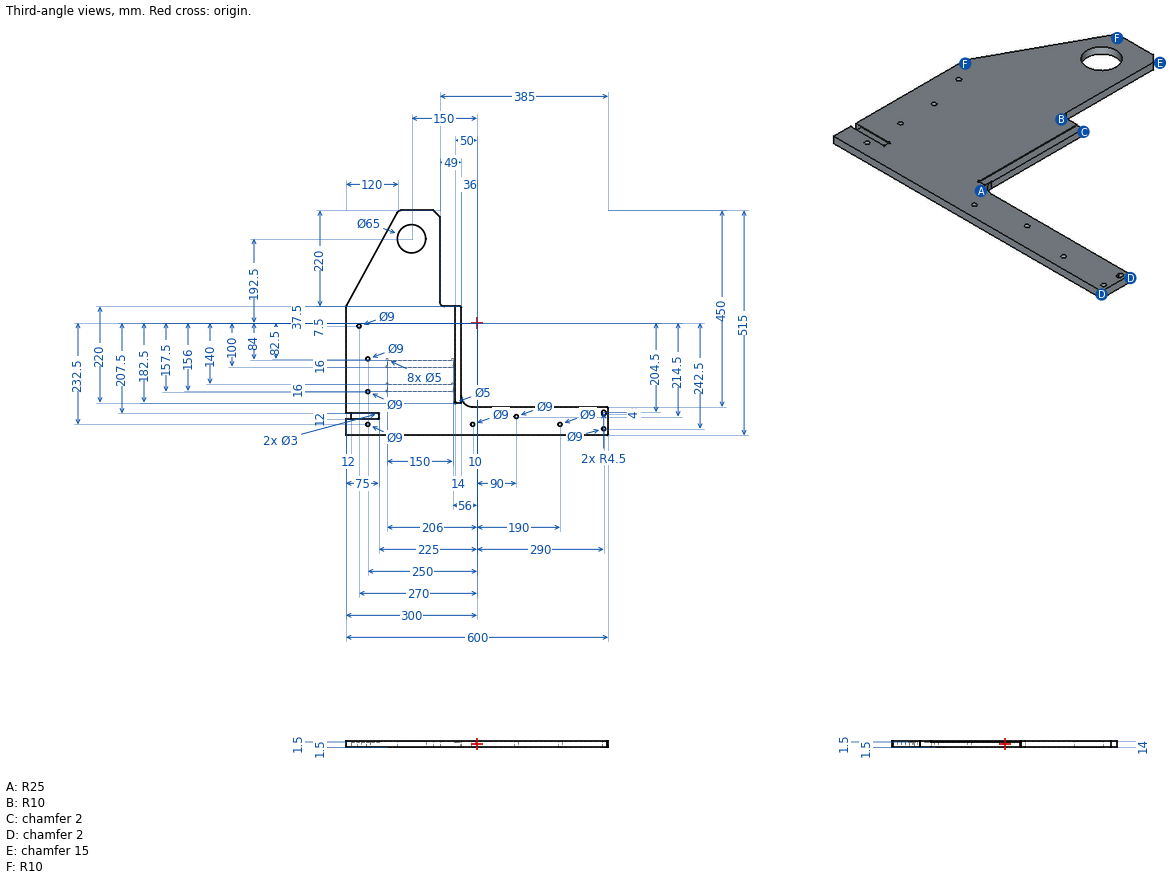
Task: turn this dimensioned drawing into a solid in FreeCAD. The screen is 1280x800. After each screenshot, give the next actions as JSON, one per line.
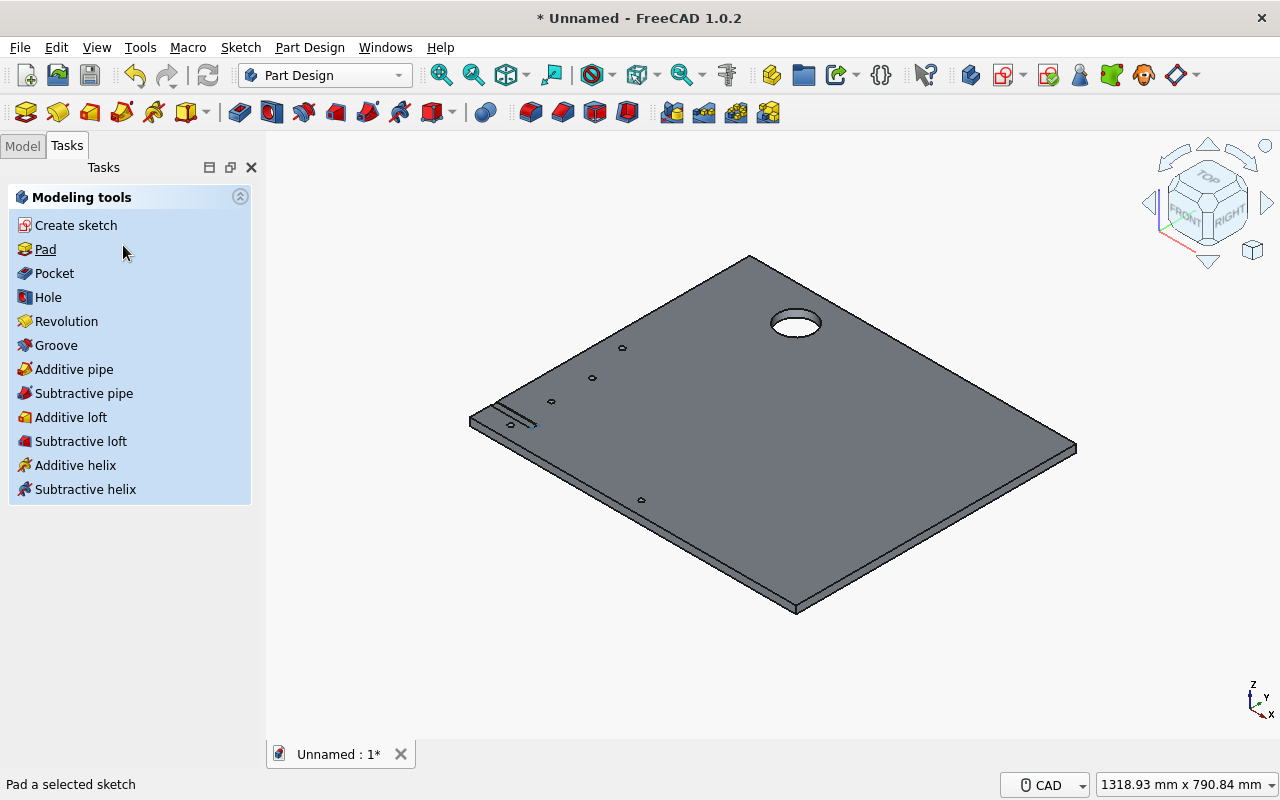
{"action": "left_click", "coordinate": [240, 112]}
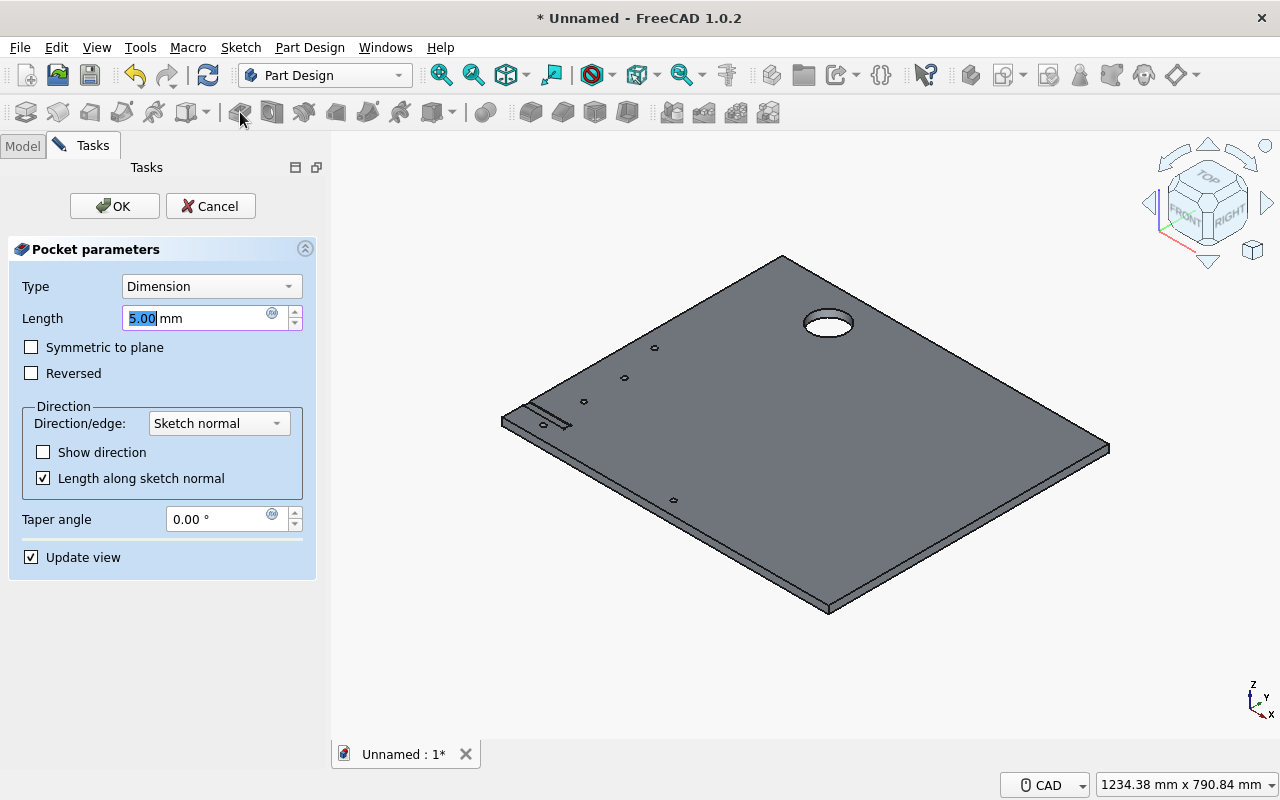
{"action": "type", "text": "1.5"}
{"action": "key", "text": "Tab"}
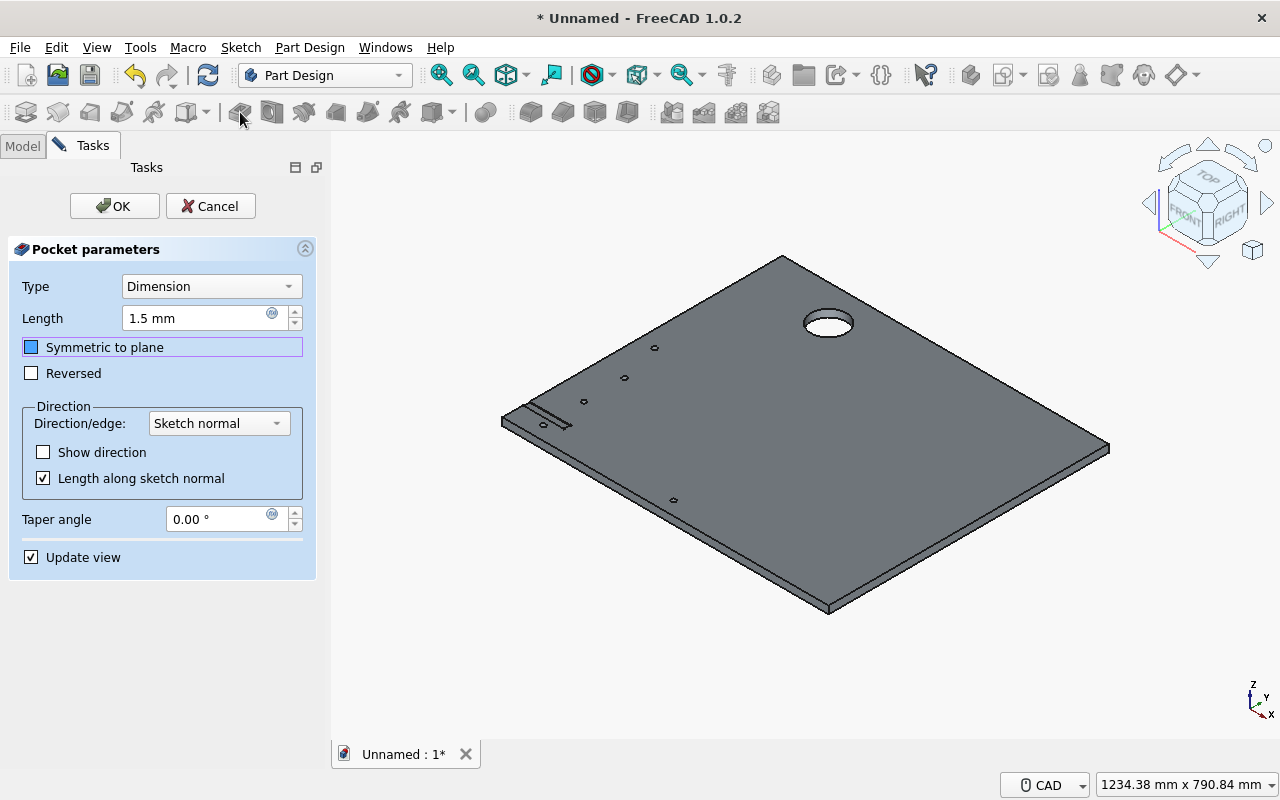
{"action": "left_click", "coordinate": [115, 206]}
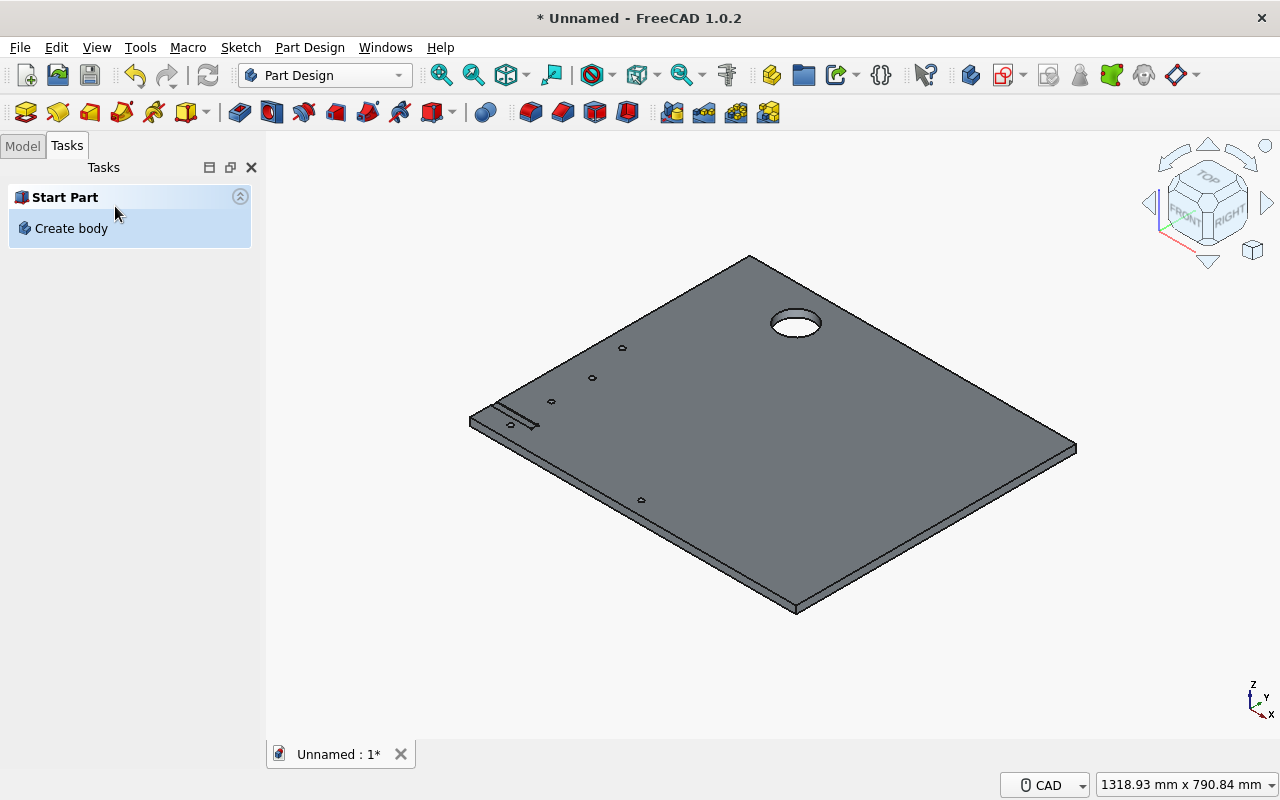
{"action": "scroll", "coordinate": [527, 422], "scroll_direction": "up", "scroll_amount": 5}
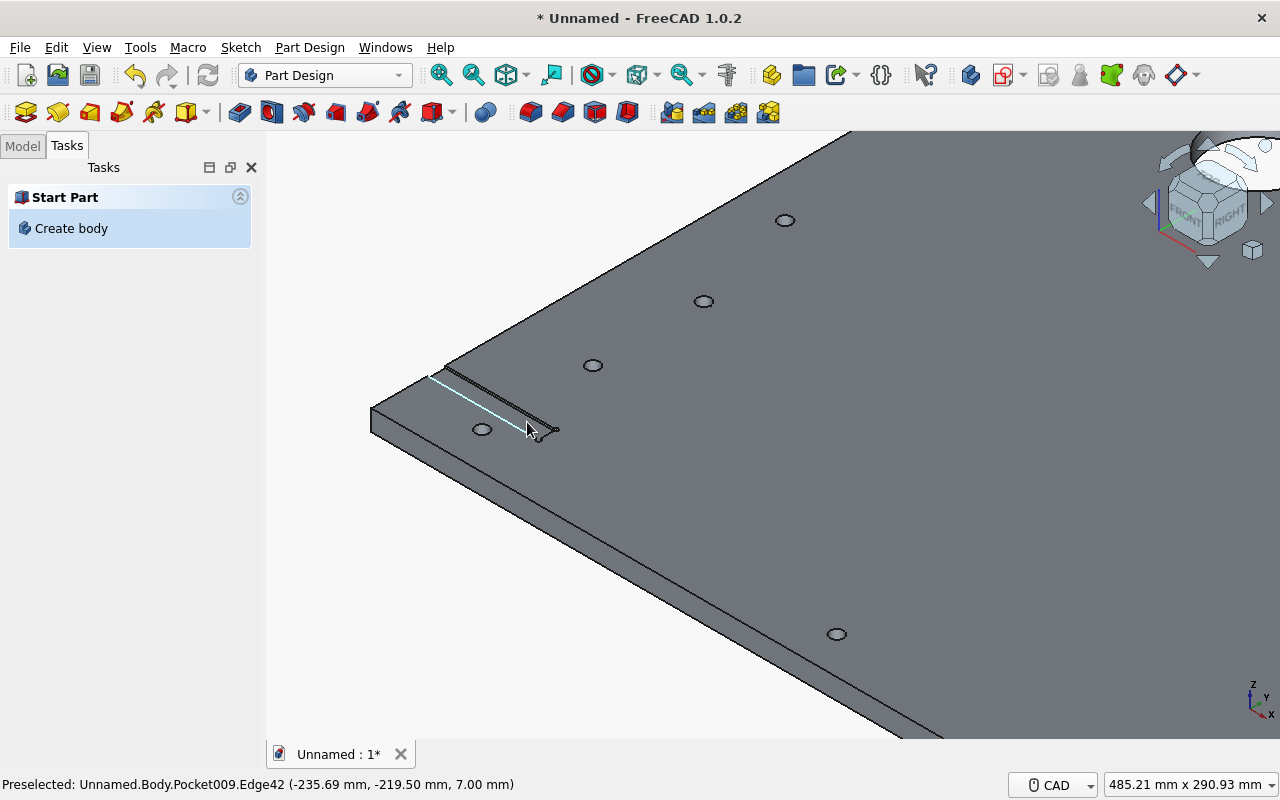
{"action": "left_click", "coordinate": [442, 76]}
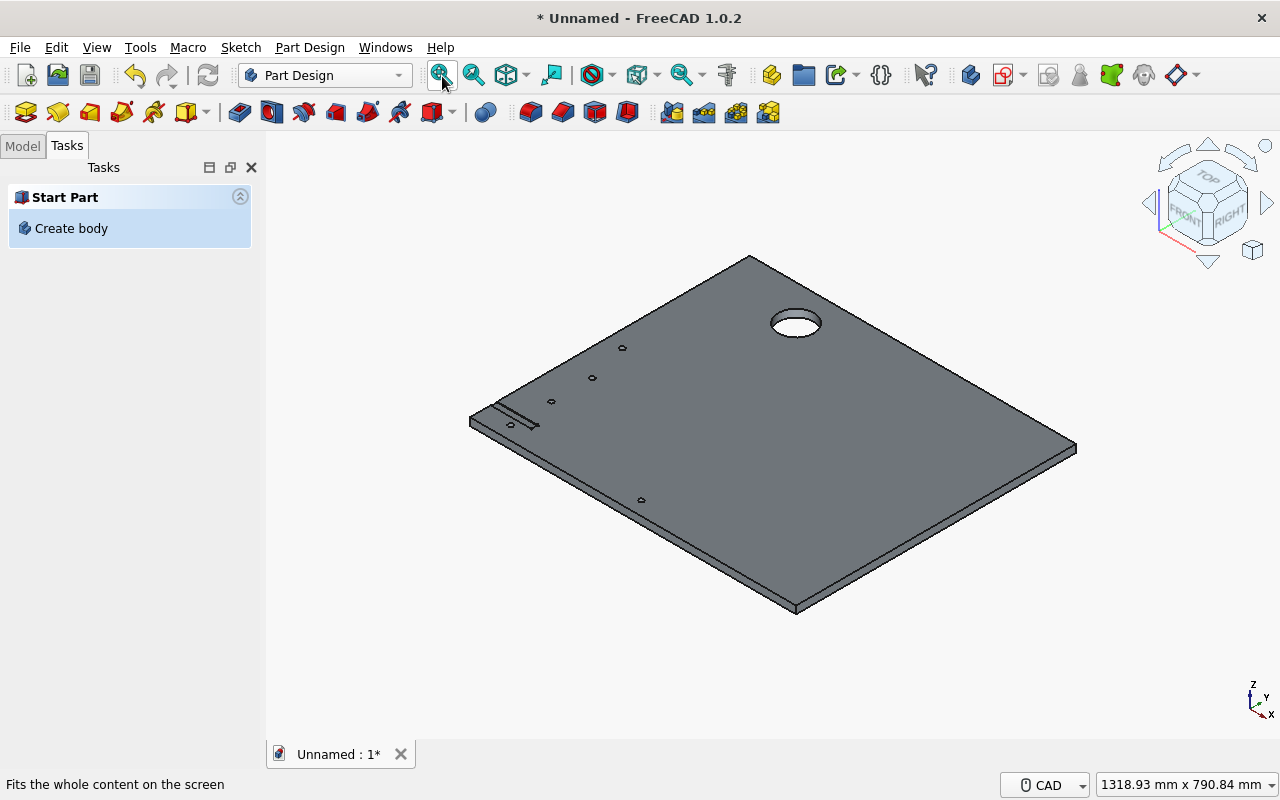
{"action": "key", "text": "2"}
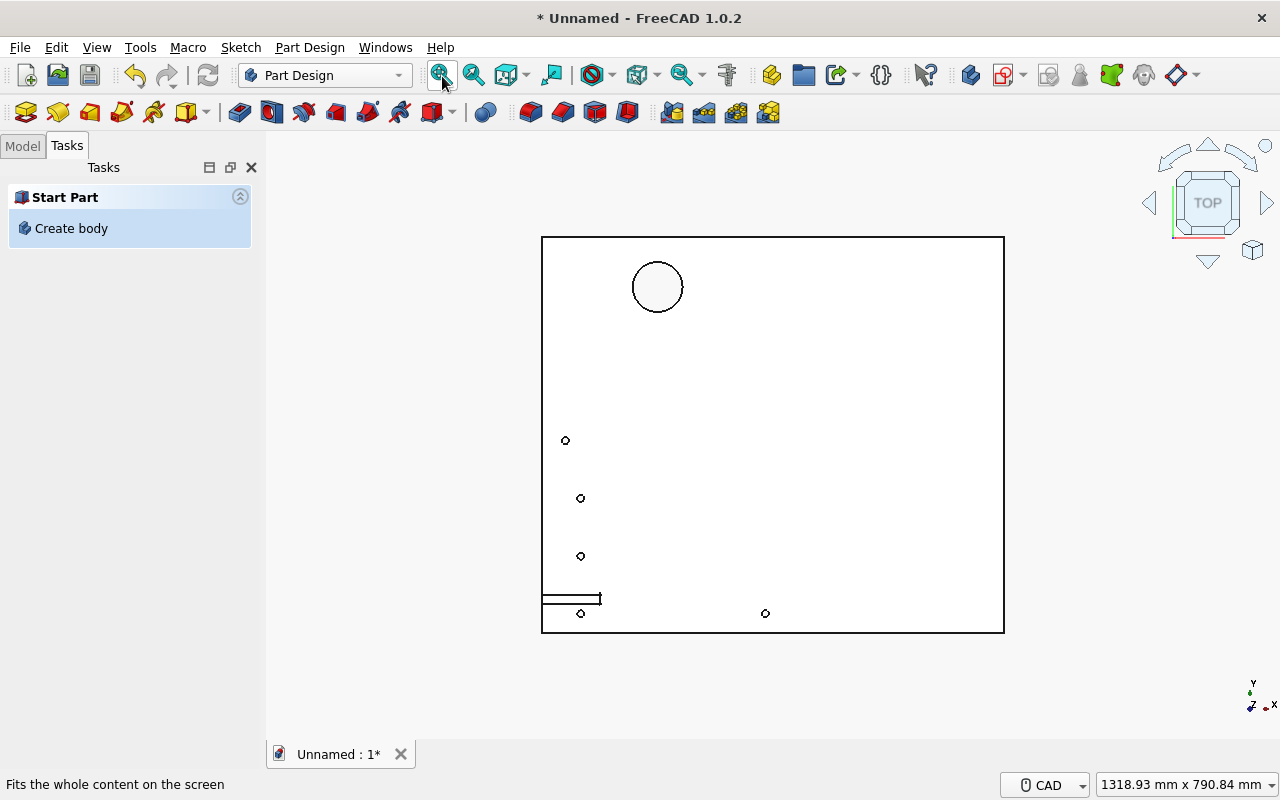
{"action": "scroll", "coordinate": [589, 598], "scroll_direction": "up", "scroll_amount": 5}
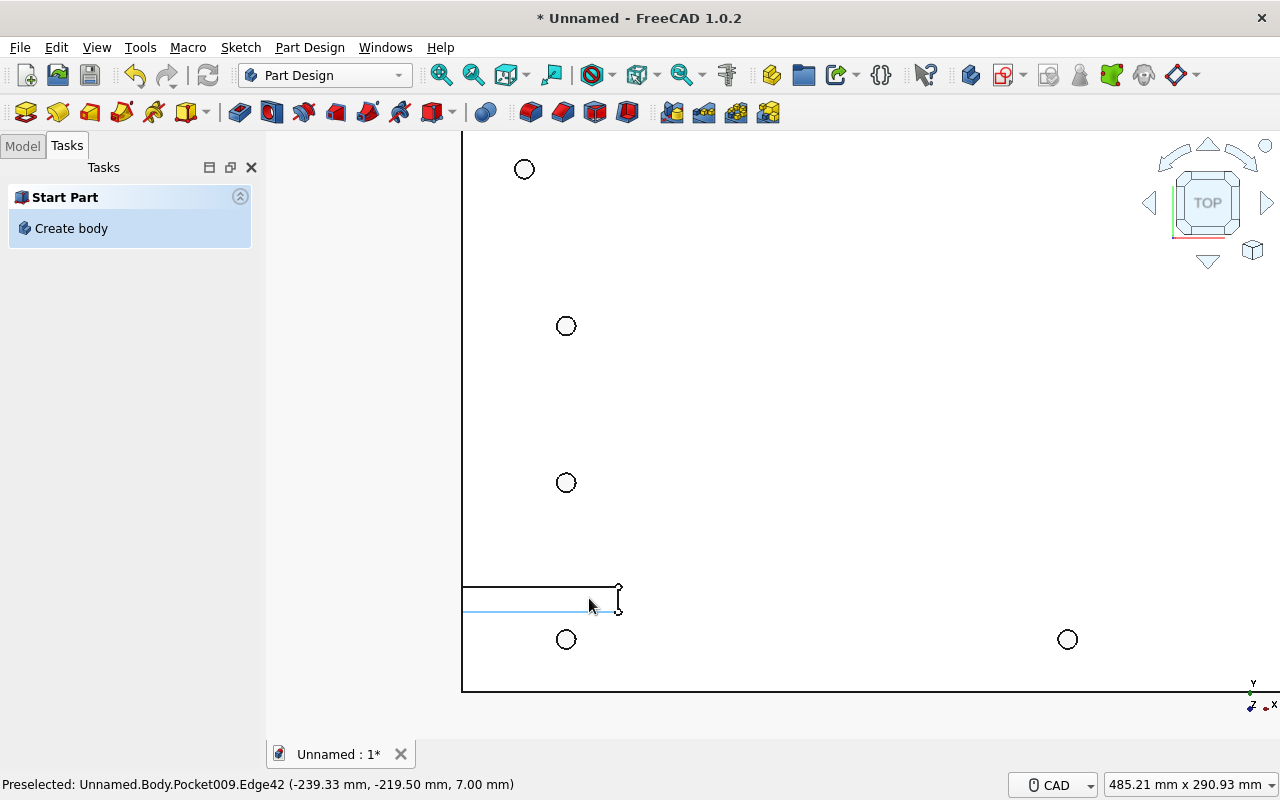
{"action": "left_click", "coordinate": [587, 599]}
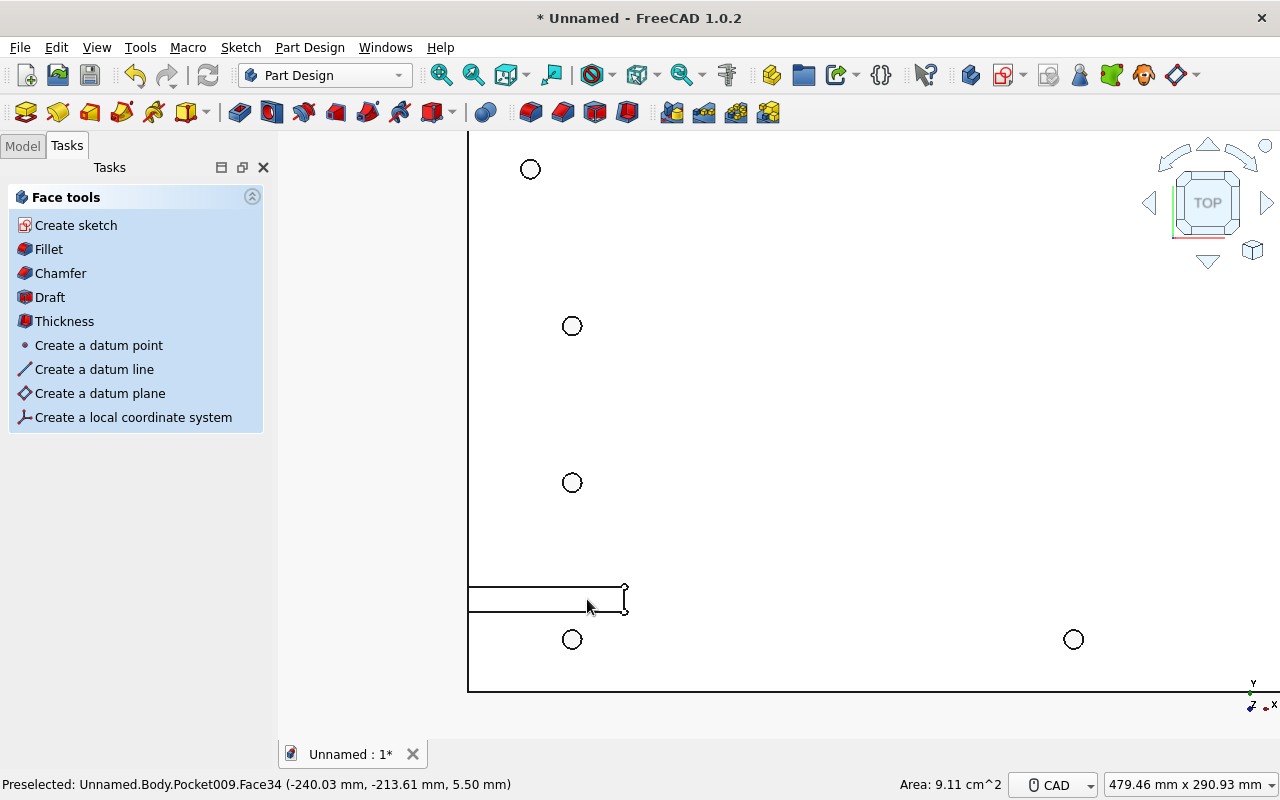
{"action": "left_click", "coordinate": [1004, 76]}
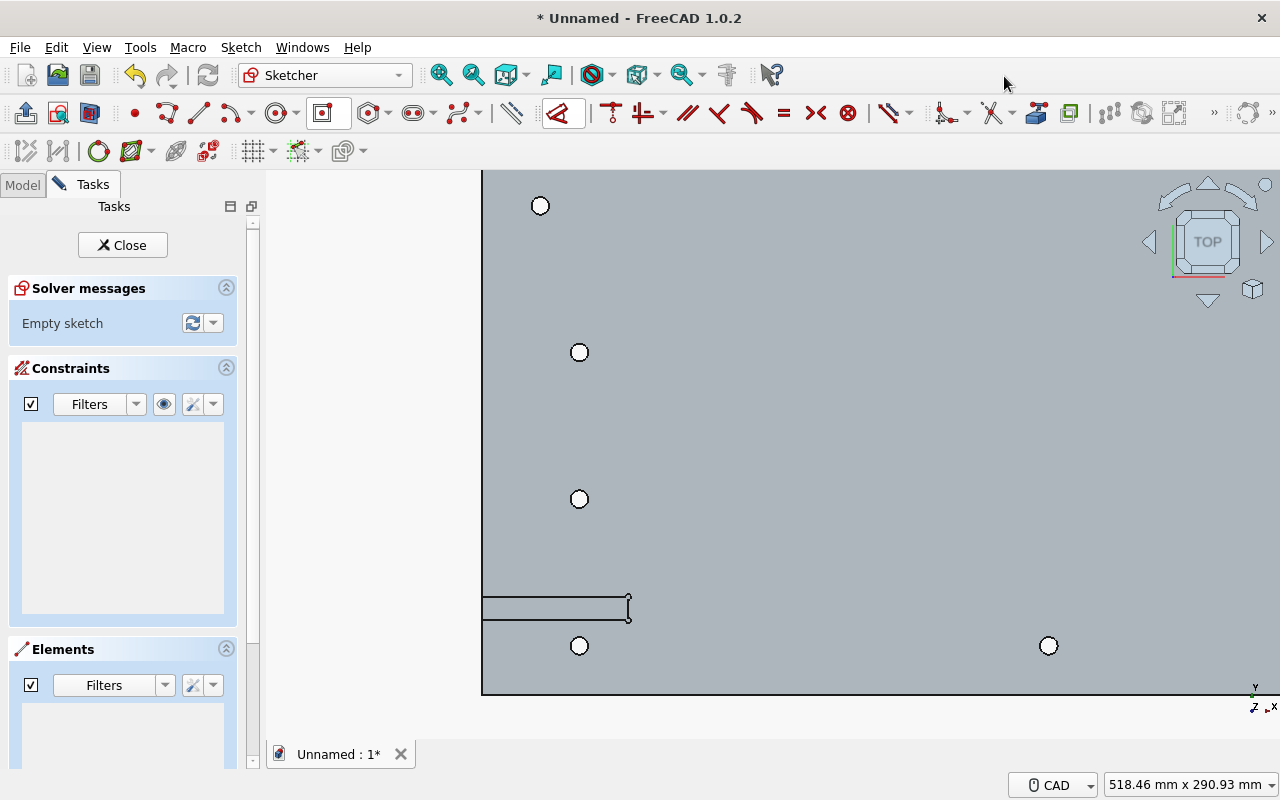
{"action": "scroll", "coordinate": [480, 619], "scroll_direction": "up", "scroll_amount": 14}